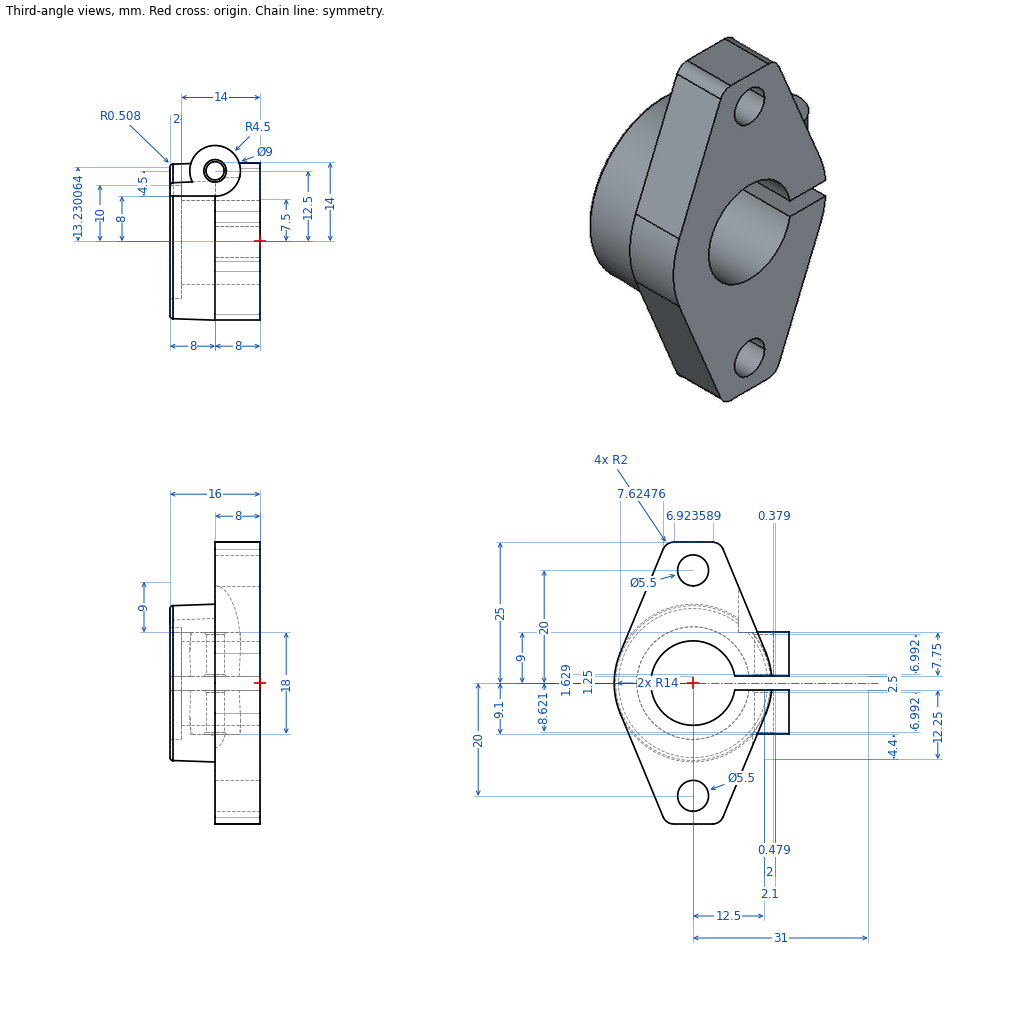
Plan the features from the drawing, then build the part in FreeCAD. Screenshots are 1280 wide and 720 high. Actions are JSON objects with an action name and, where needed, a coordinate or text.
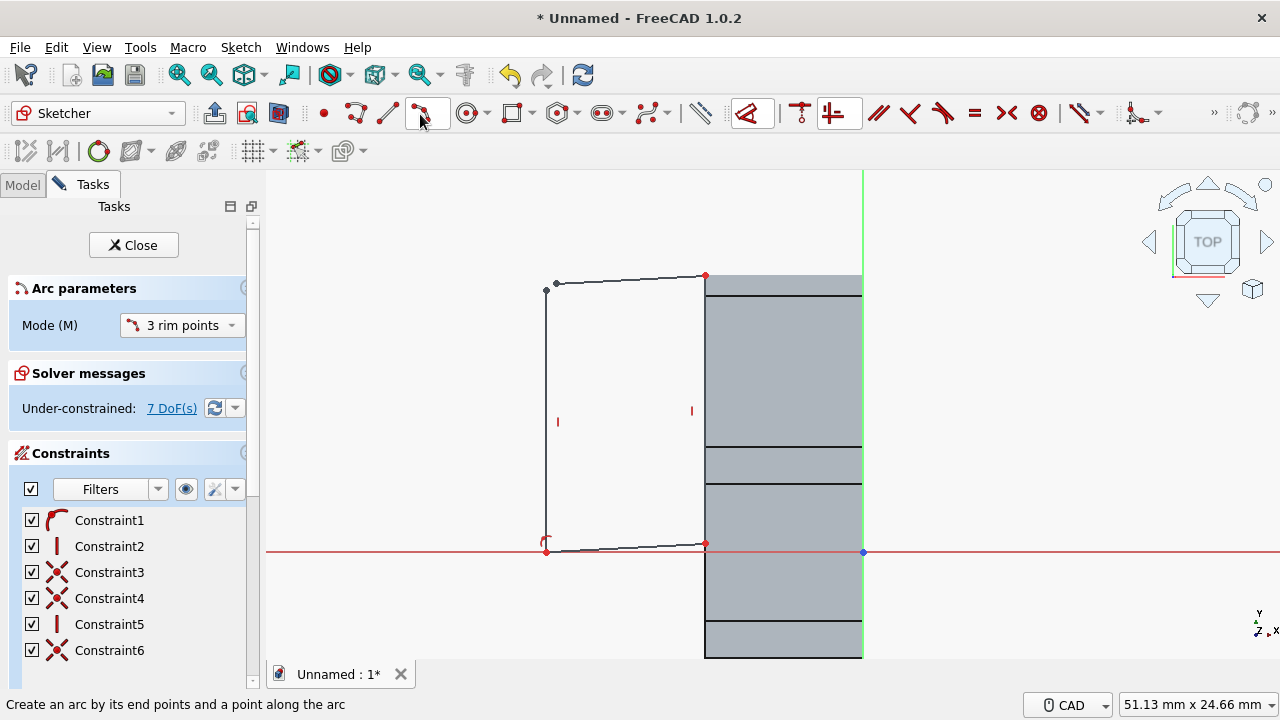
{"action": "left_click", "coordinate": [556, 284]}
{"action": "left_click", "coordinate": [546, 291]}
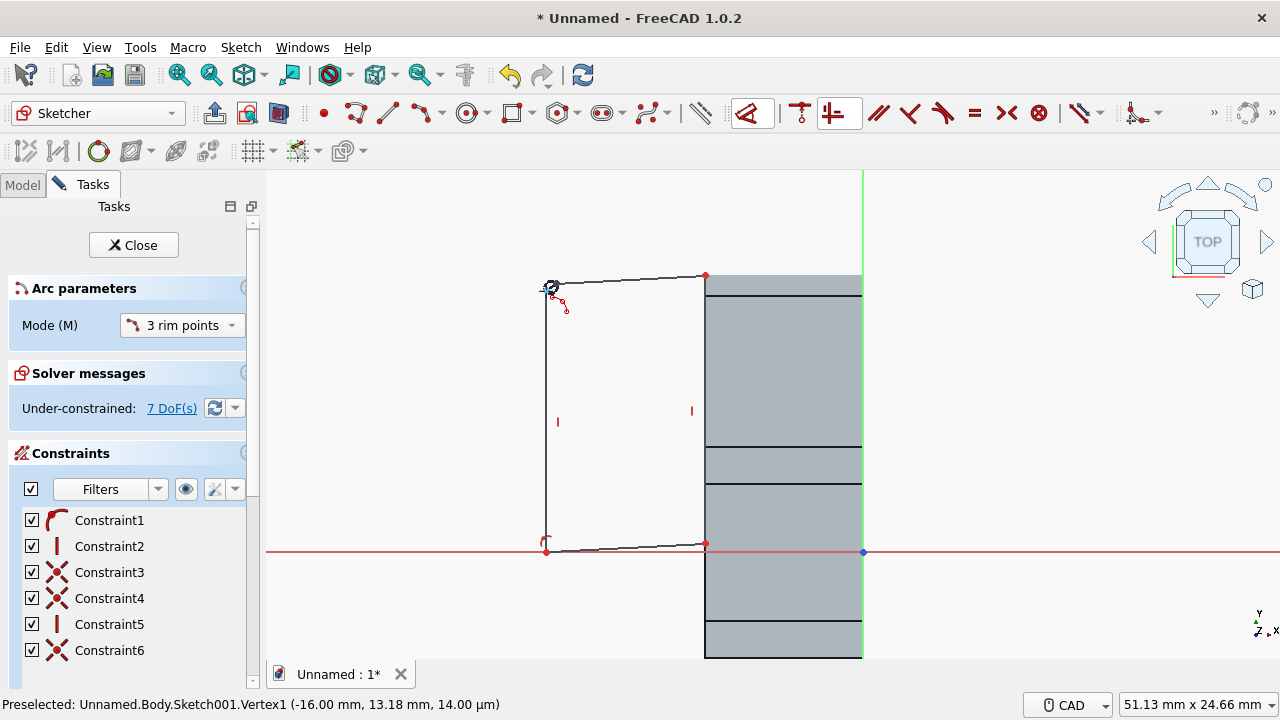
{"action": "scroll", "coordinate": [549, 283], "scroll_direction": "up", "scroll_amount": 9}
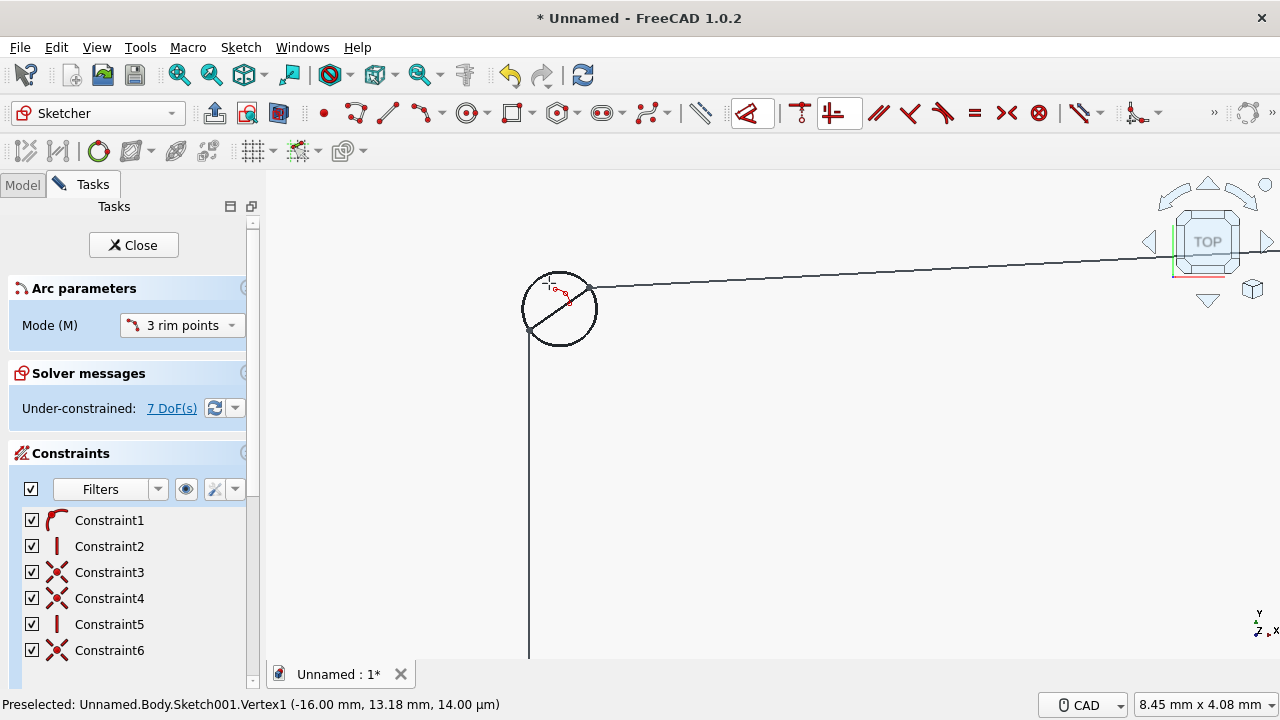
{"action": "left_click", "coordinate": [546, 281]}
{"action": "key", "text": "Escape"}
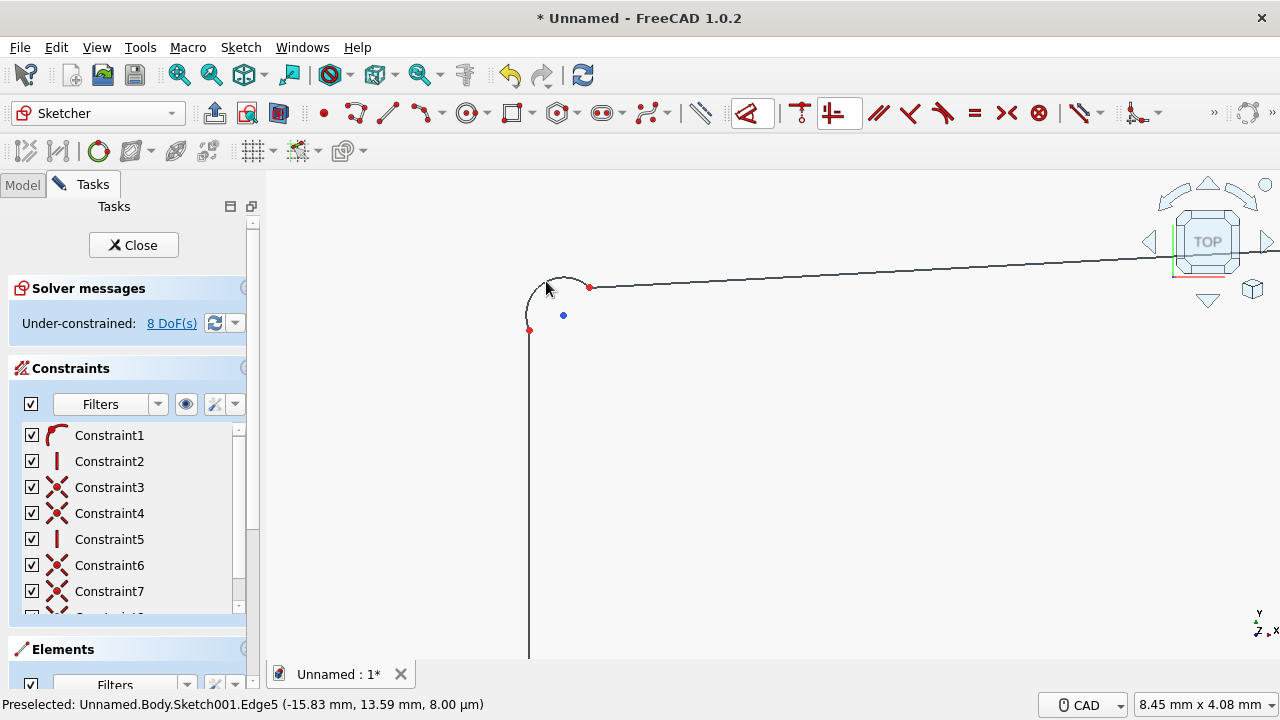
{"action": "scroll", "coordinate": [549, 284], "scroll_direction": "down", "scroll_amount": 9}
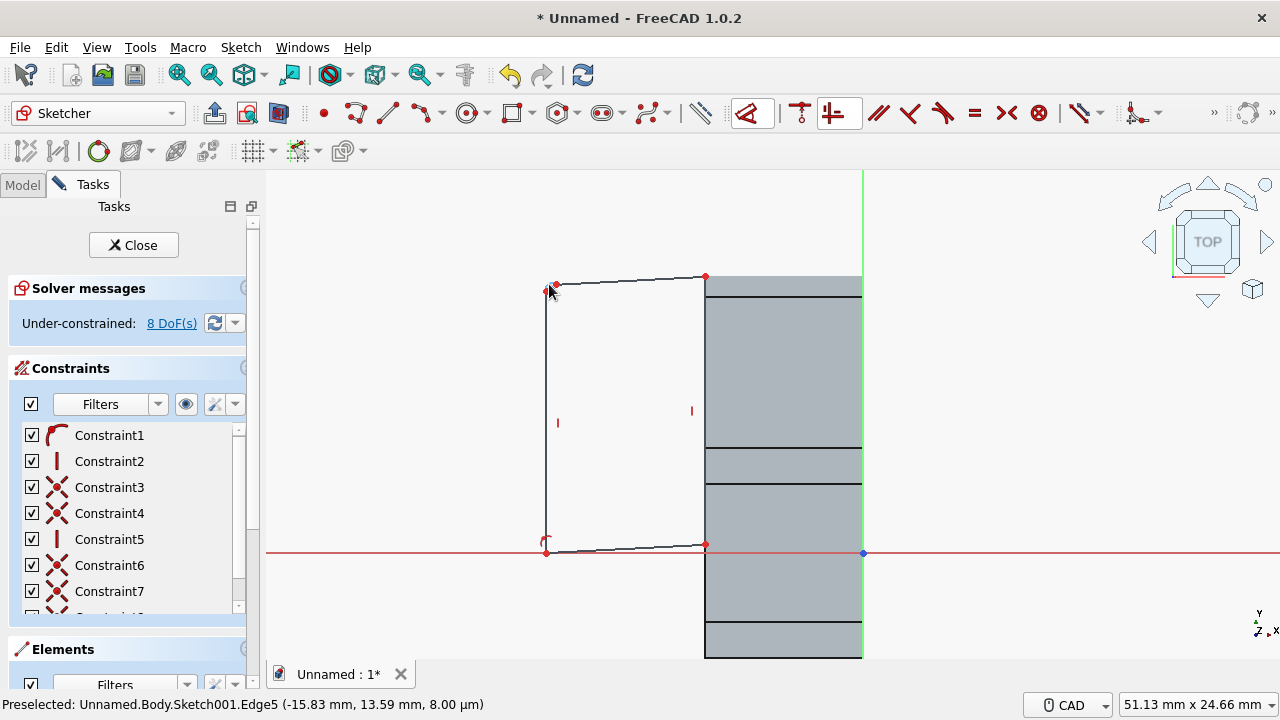
{"action": "left_click", "coordinate": [546, 370]}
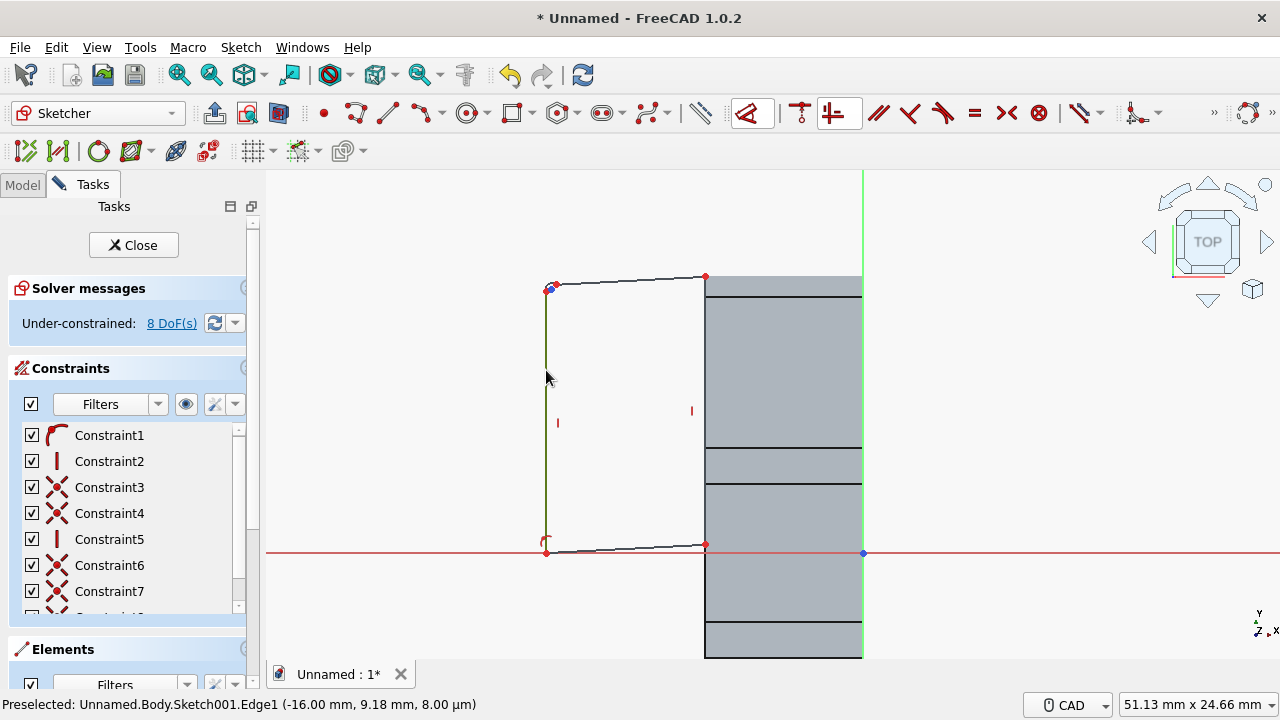
{"action": "scroll", "coordinate": [548, 284], "scroll_direction": "up", "scroll_amount": 4}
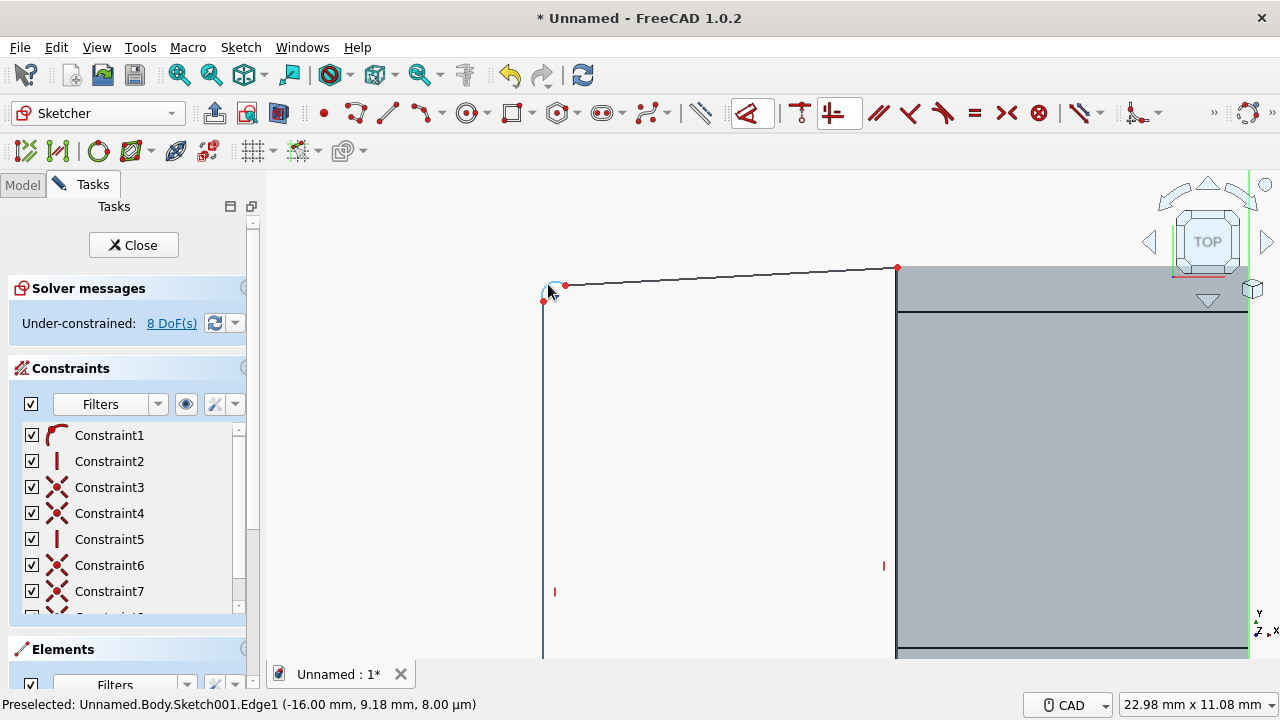
{"action": "left_click", "coordinate": [548, 284]}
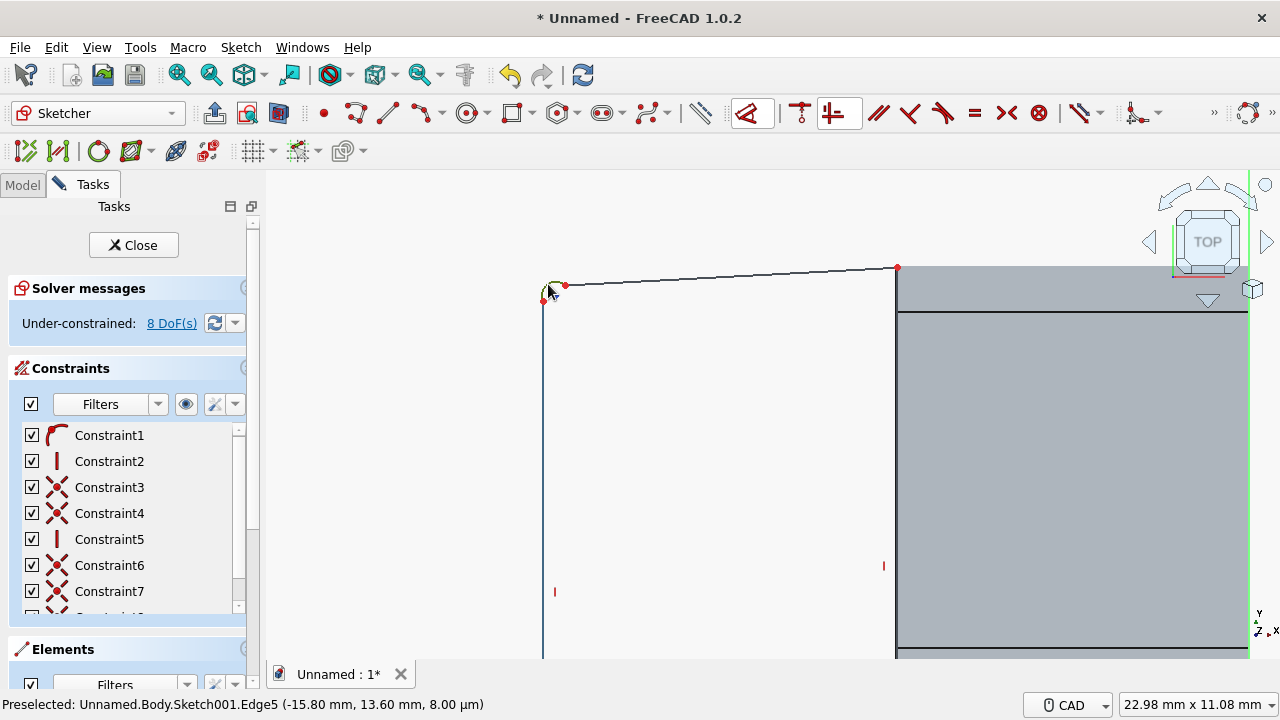
{"action": "key", "text": "t"}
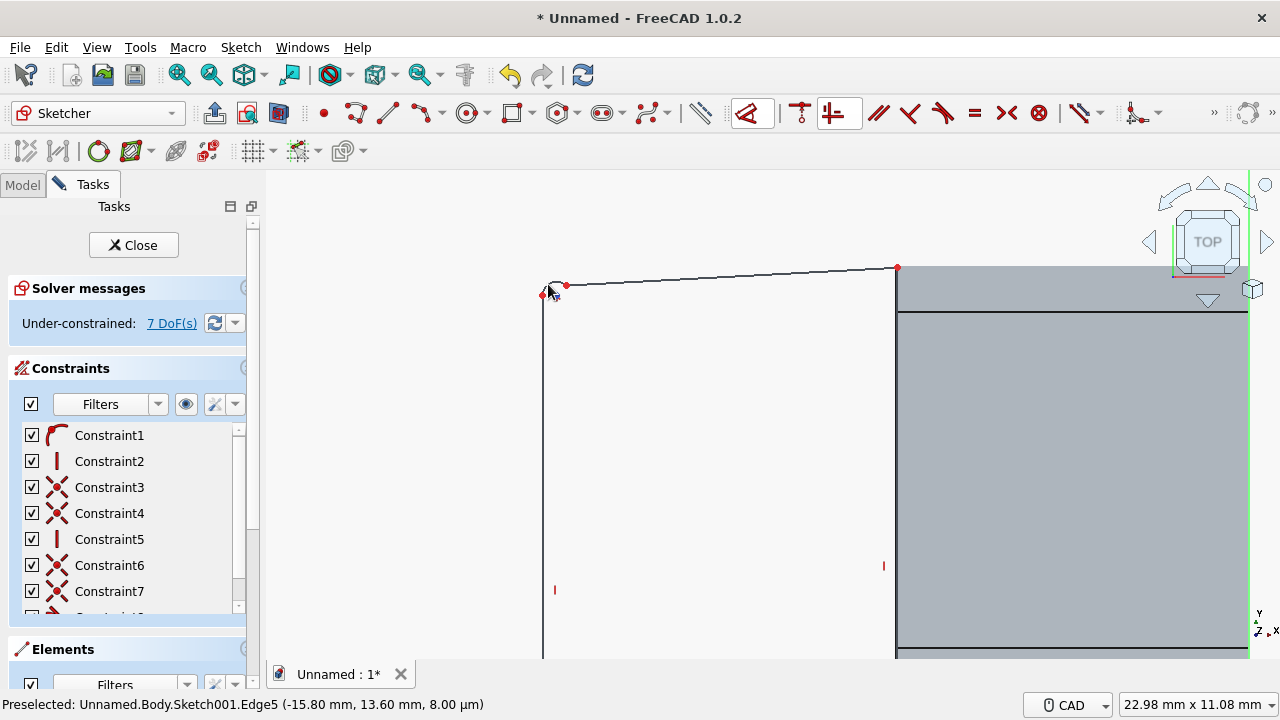
{"action": "left_click", "coordinate": [798, 273]}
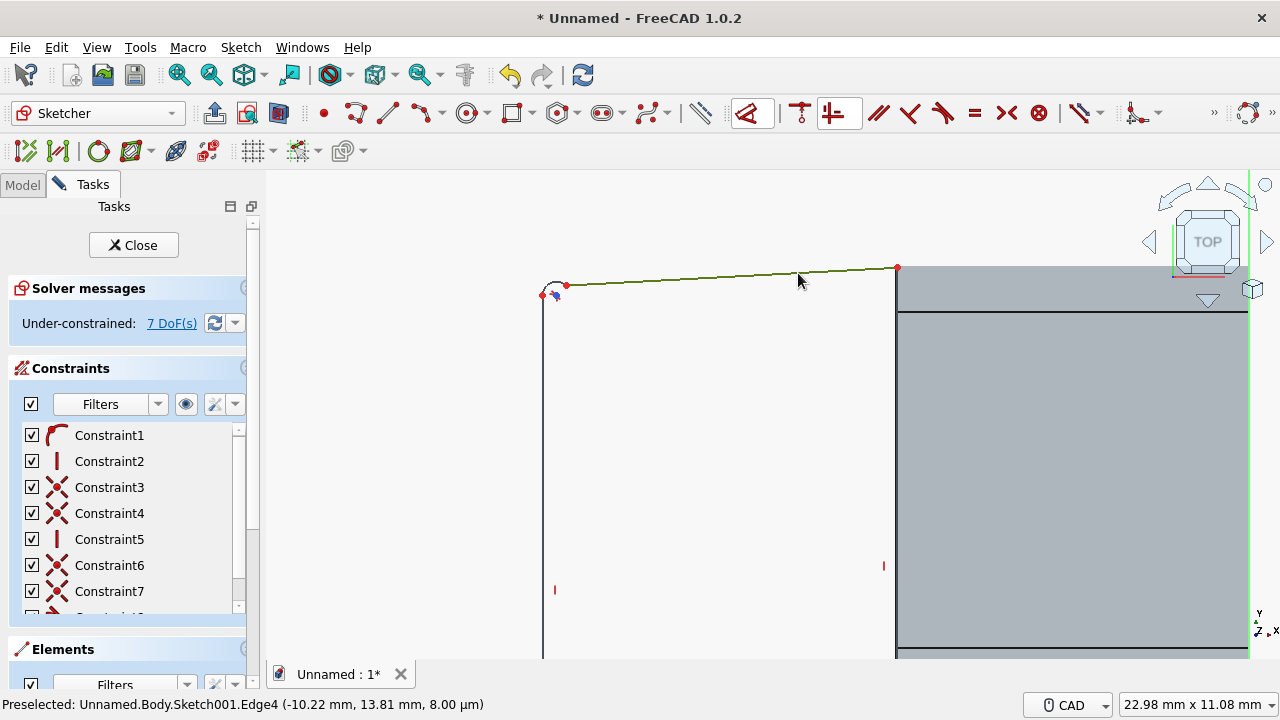
{"action": "scroll", "coordinate": [558, 282], "scroll_direction": "up", "scroll_amount": 2}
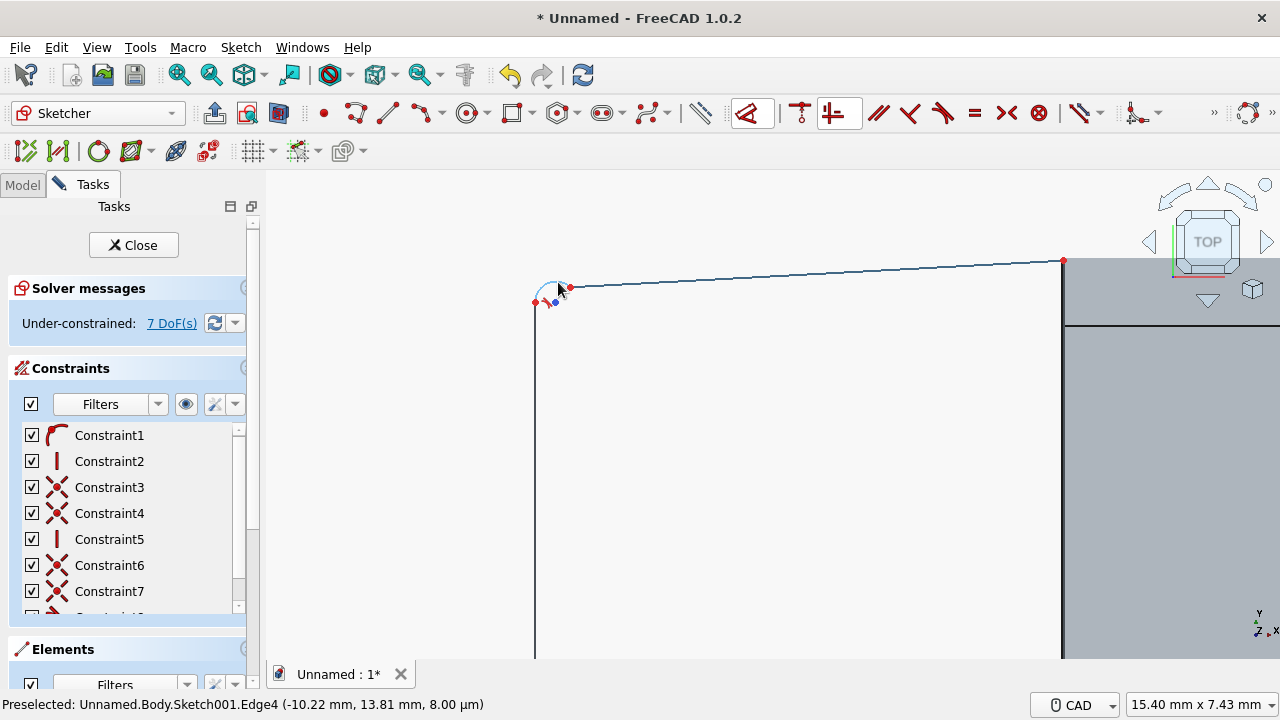
{"action": "left_click", "coordinate": [557, 282]}